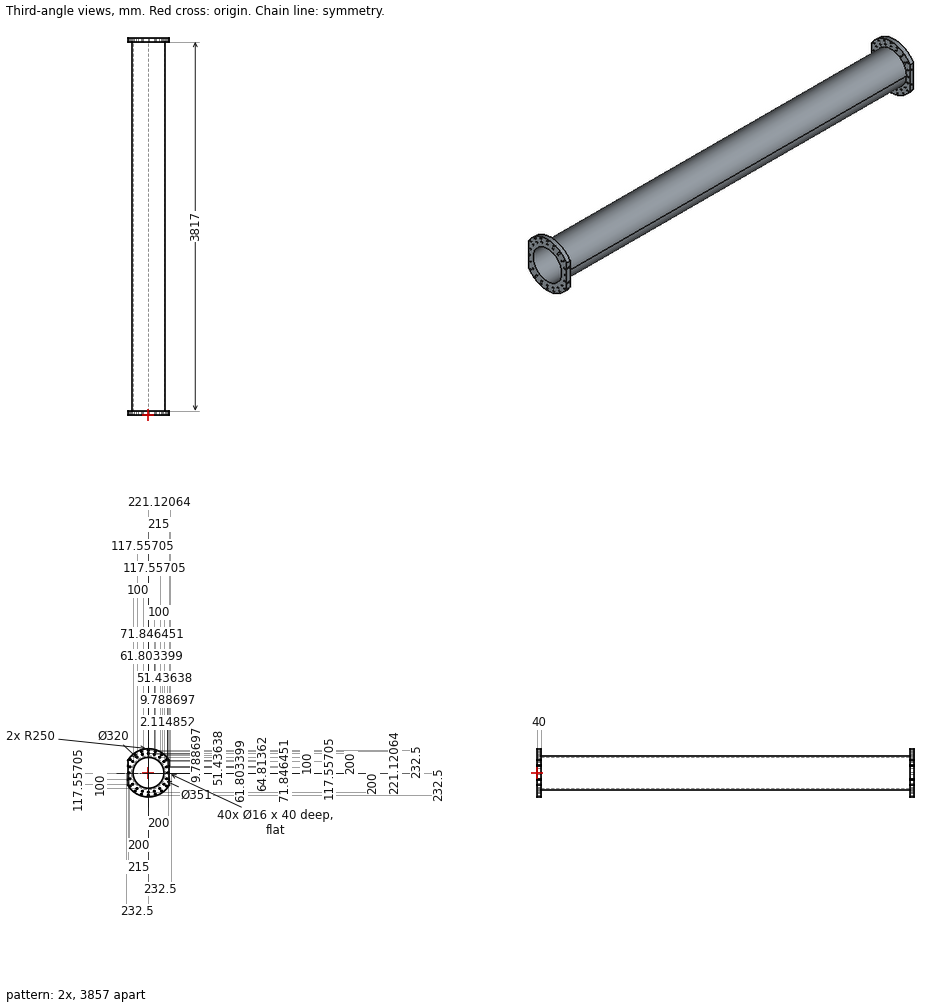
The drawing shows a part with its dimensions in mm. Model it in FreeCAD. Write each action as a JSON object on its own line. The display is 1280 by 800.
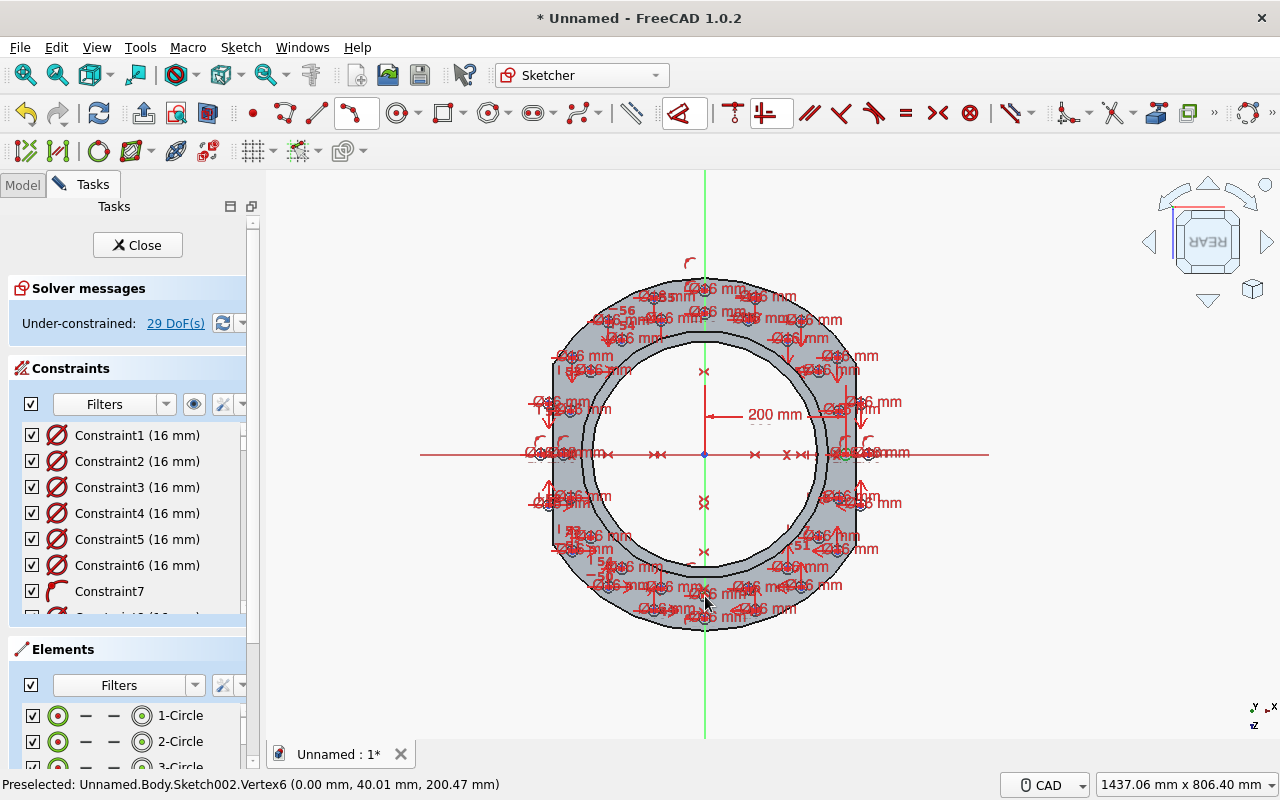
{"action": "left_click", "coordinate": [702, 114]}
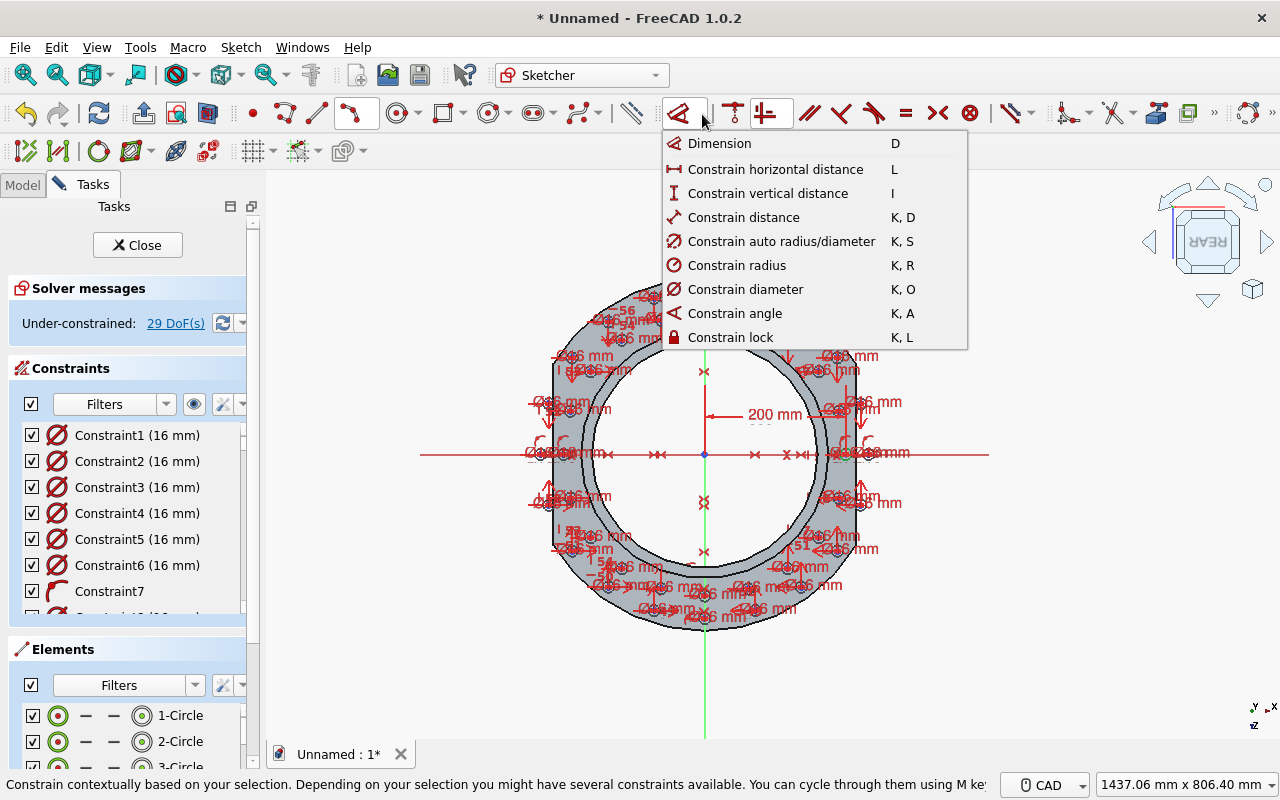
{"action": "left_click", "coordinate": [815, 193]}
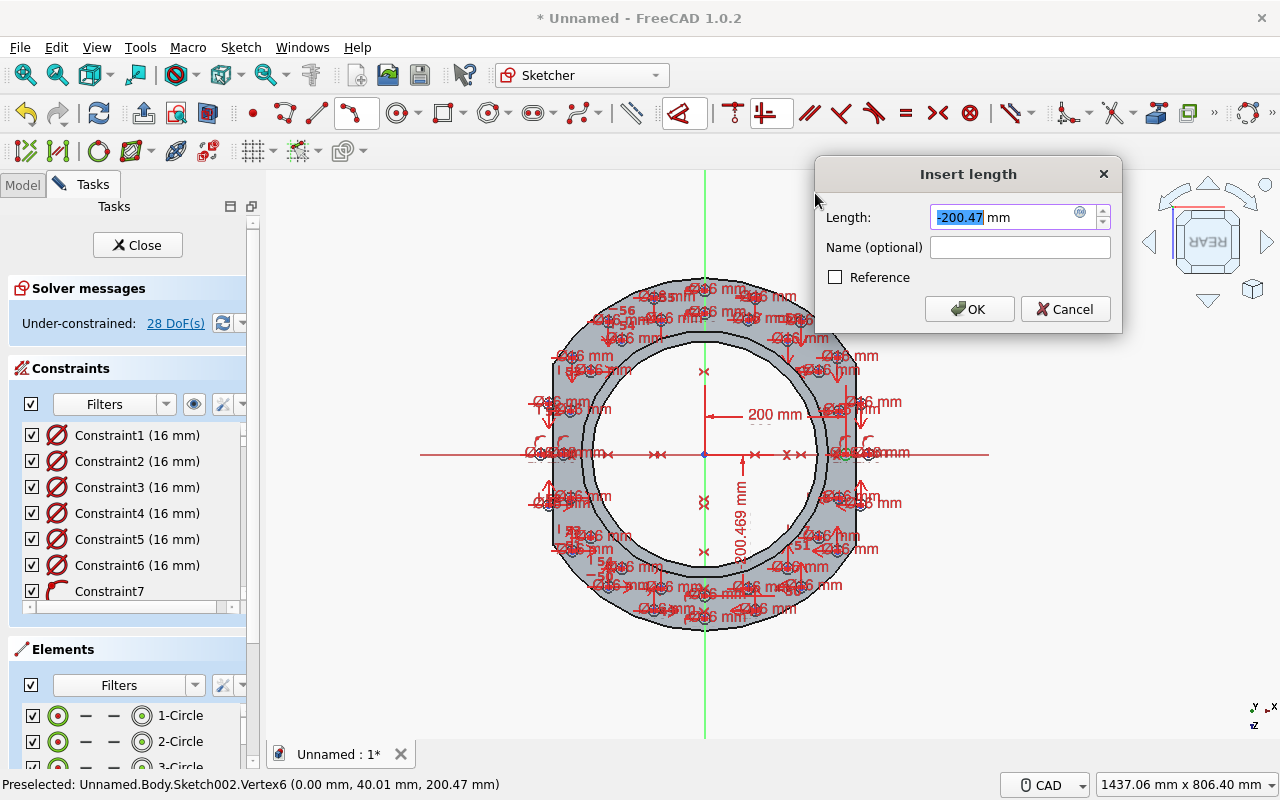
{"action": "type", "text": "-200"}
{"action": "key", "text": "Return"}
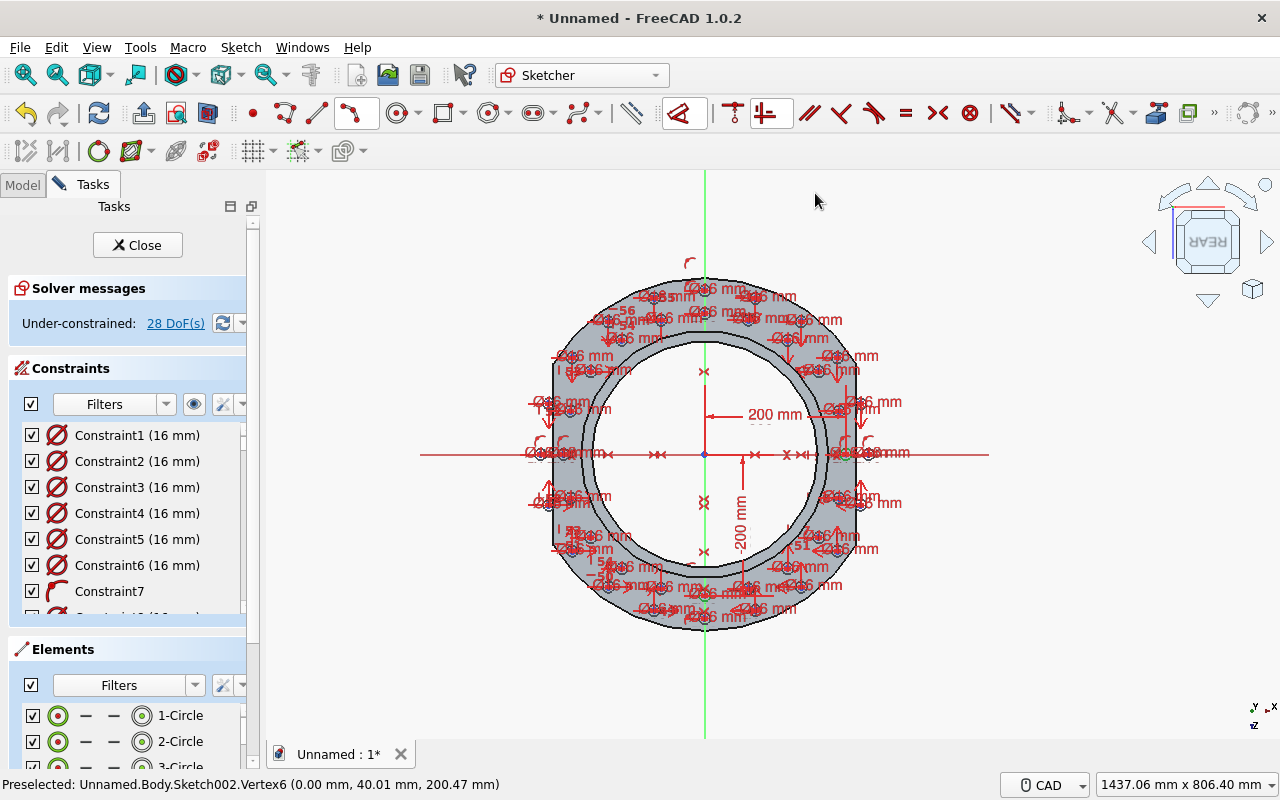
{"action": "left_click", "coordinate": [564, 454]}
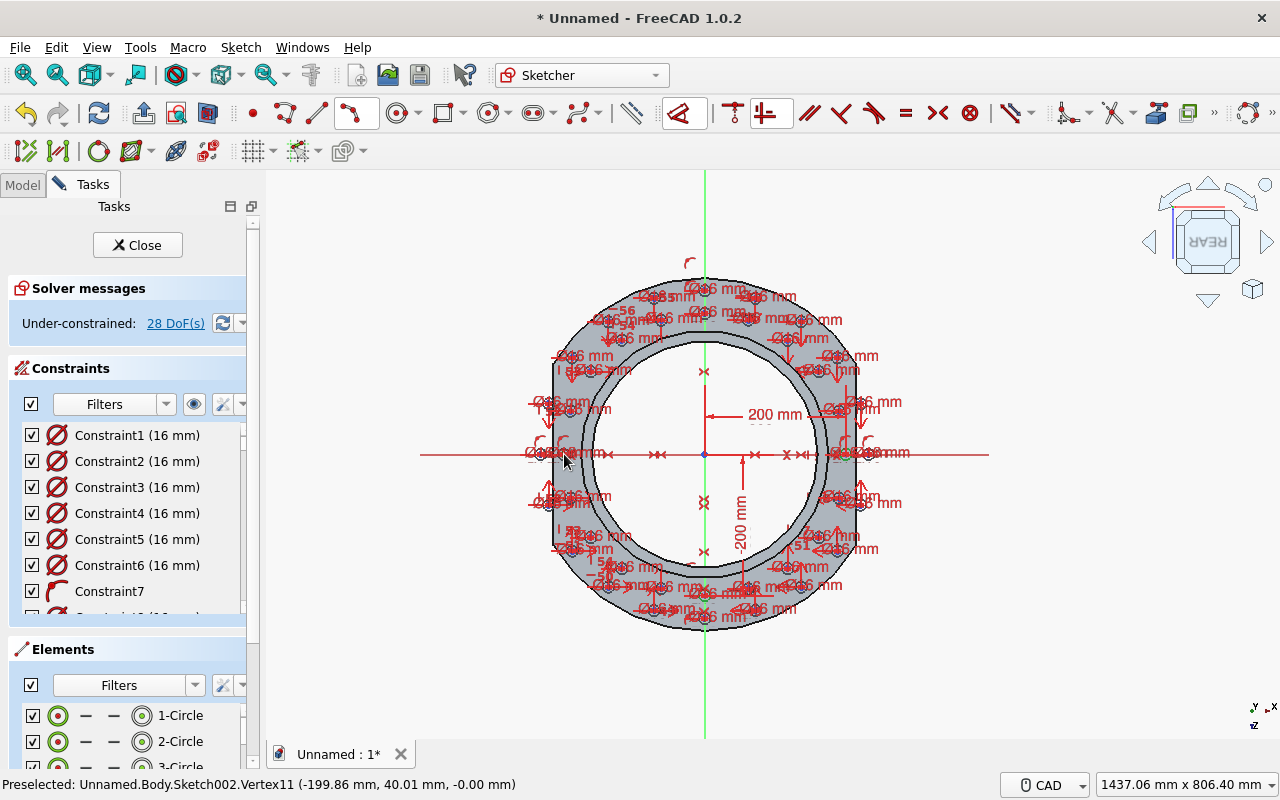
{"action": "left_click", "coordinate": [702, 114]}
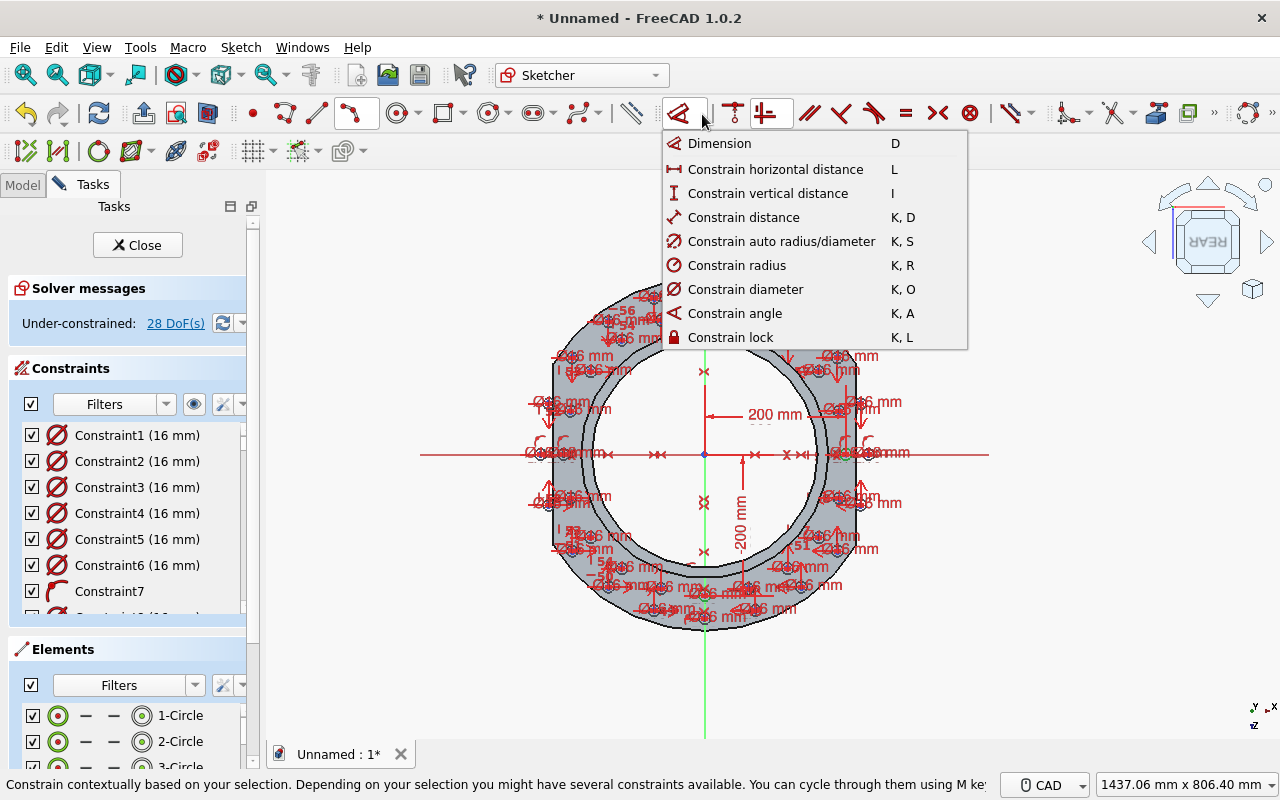
{"action": "left_click", "coordinate": [815, 169]}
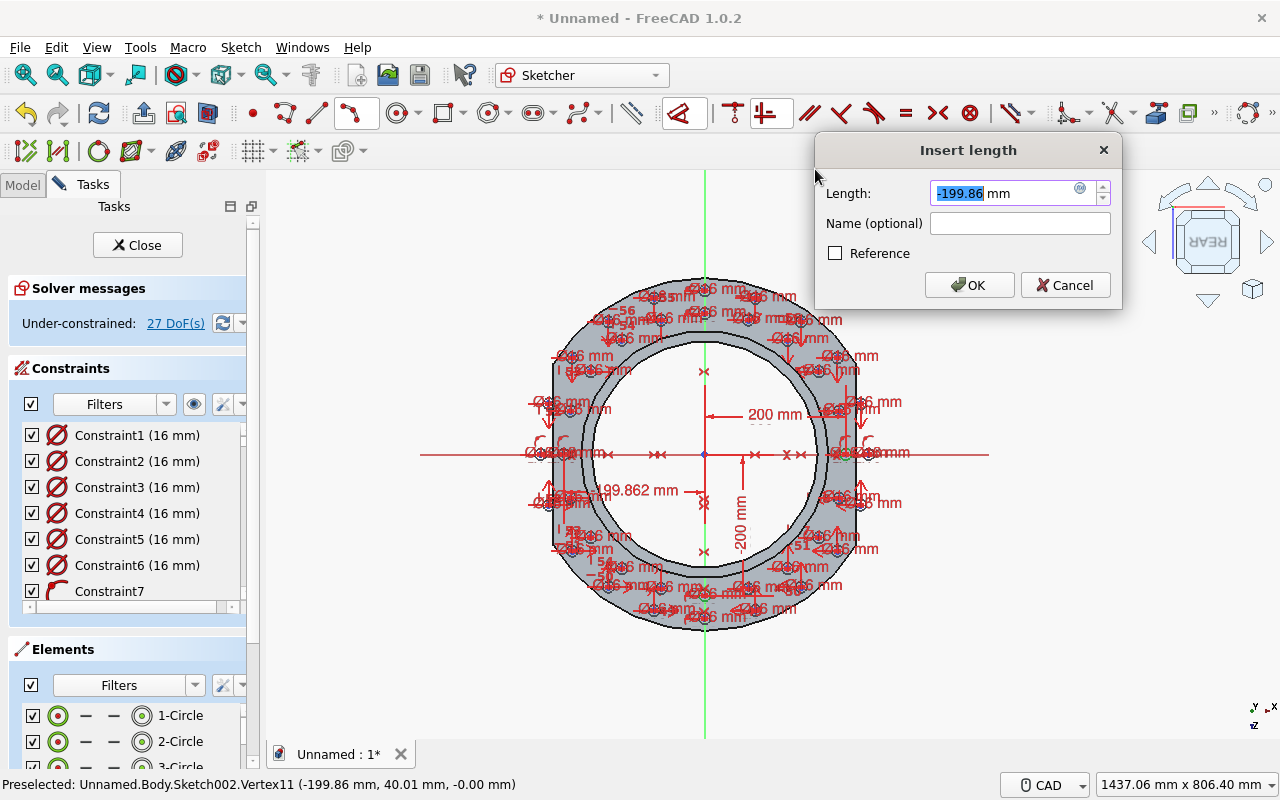
{"action": "type", "text": "-200"}
{"action": "key", "text": "Return"}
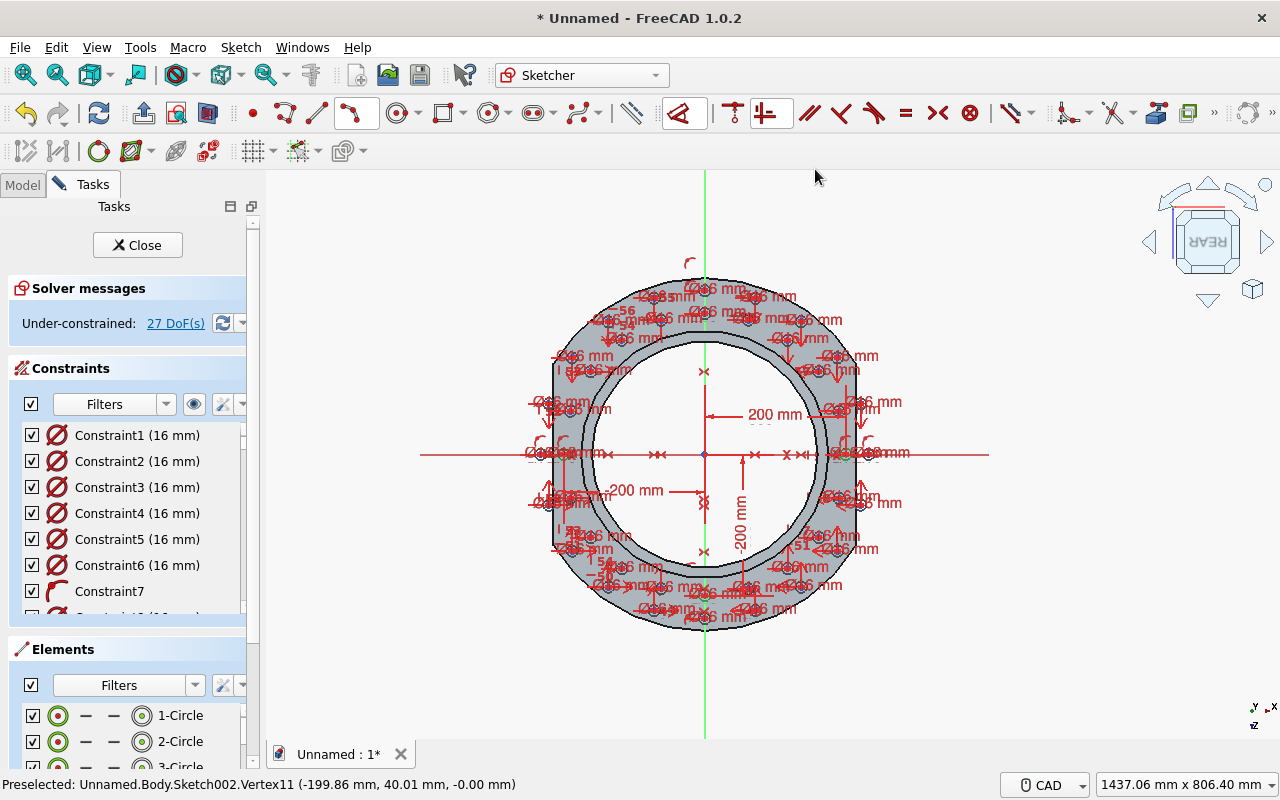
{"action": "left_click", "coordinate": [705, 314]}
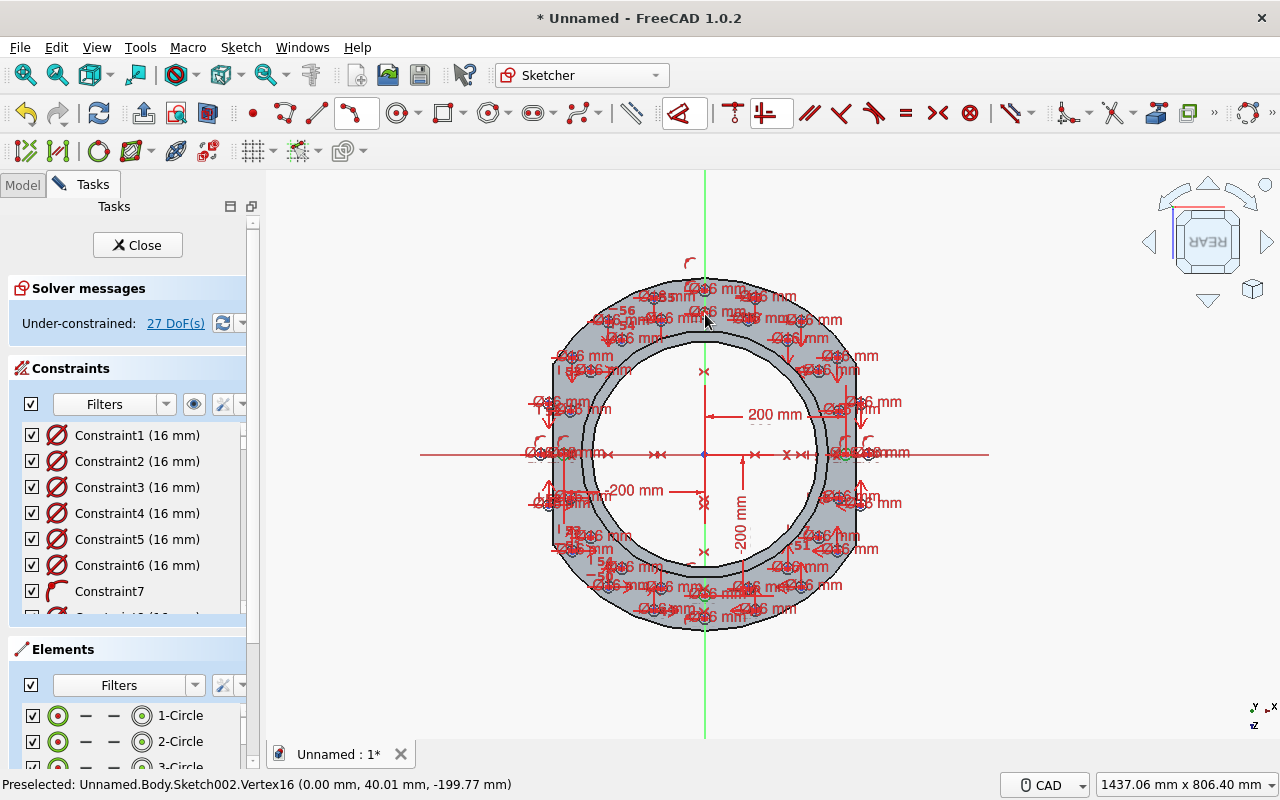
{"action": "left_click", "coordinate": [702, 114]}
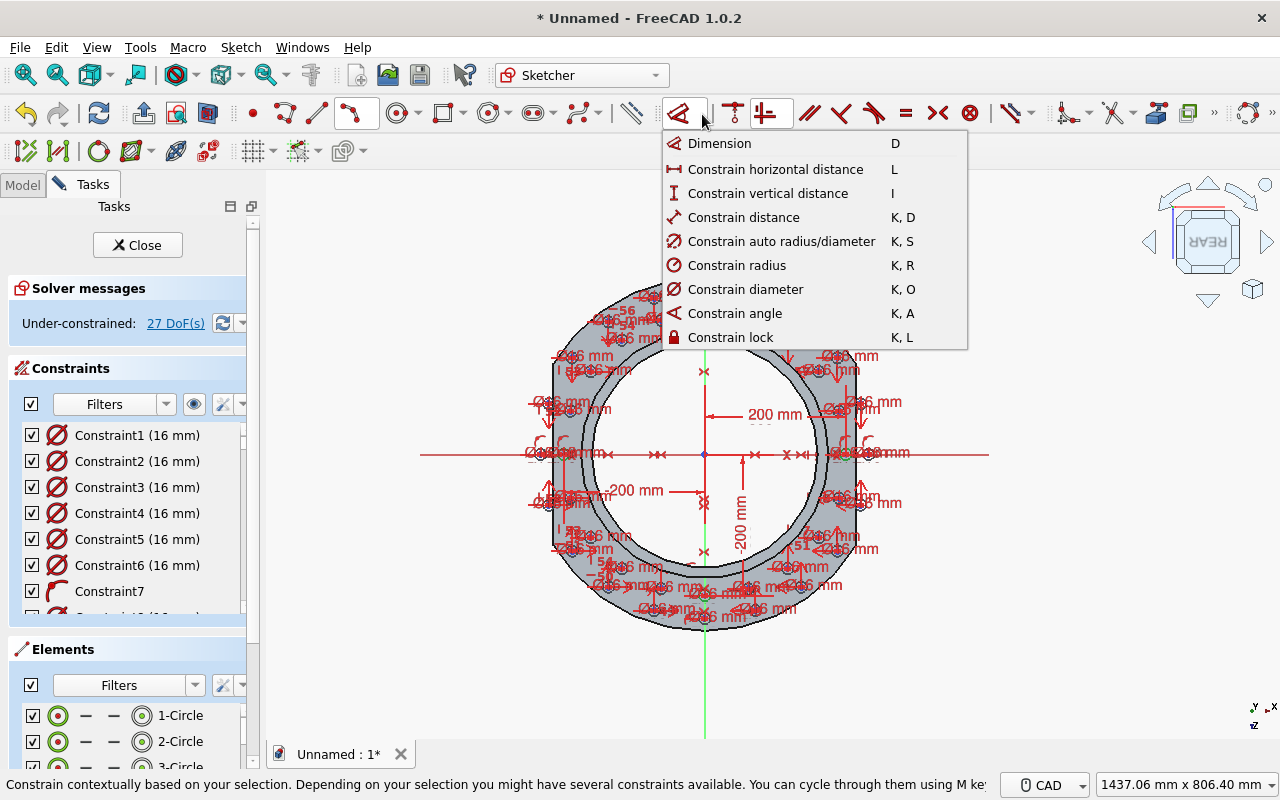
{"action": "left_click", "coordinate": [815, 193]}